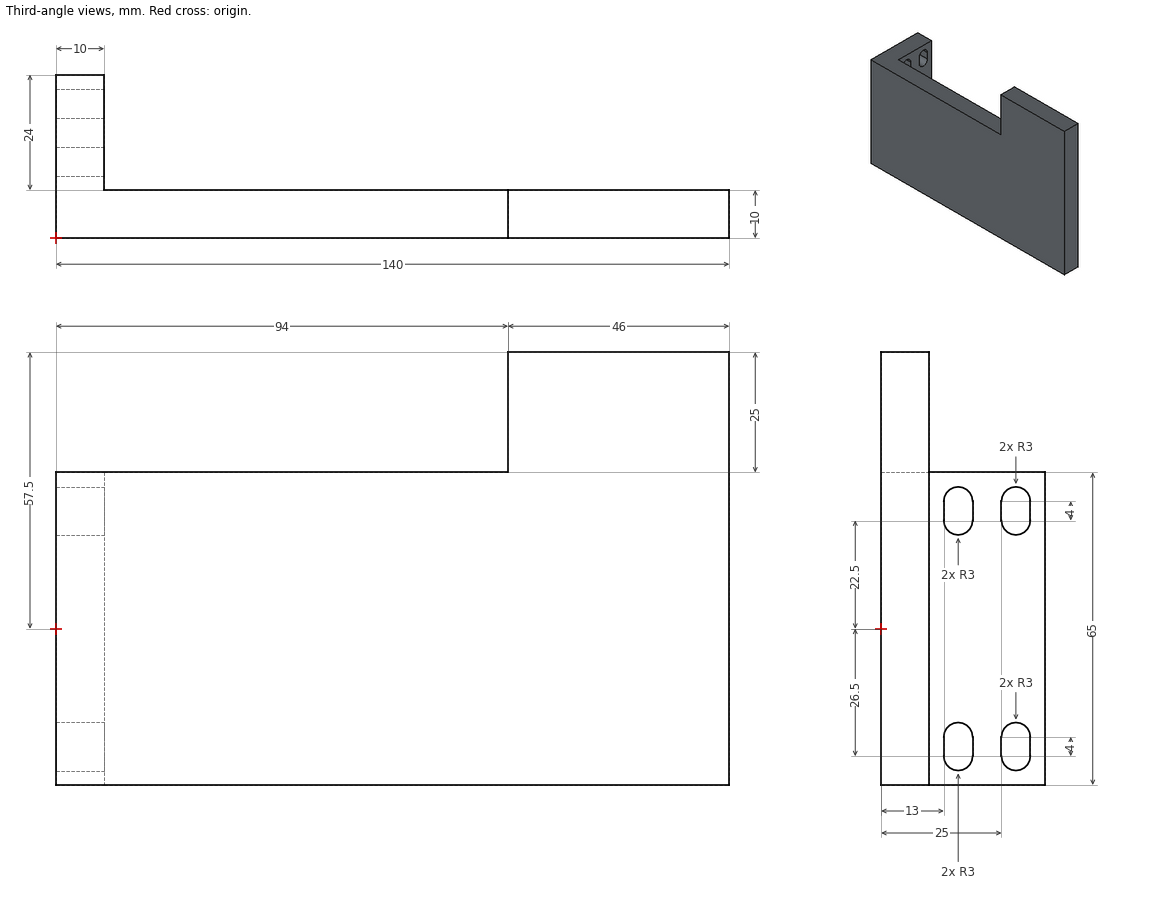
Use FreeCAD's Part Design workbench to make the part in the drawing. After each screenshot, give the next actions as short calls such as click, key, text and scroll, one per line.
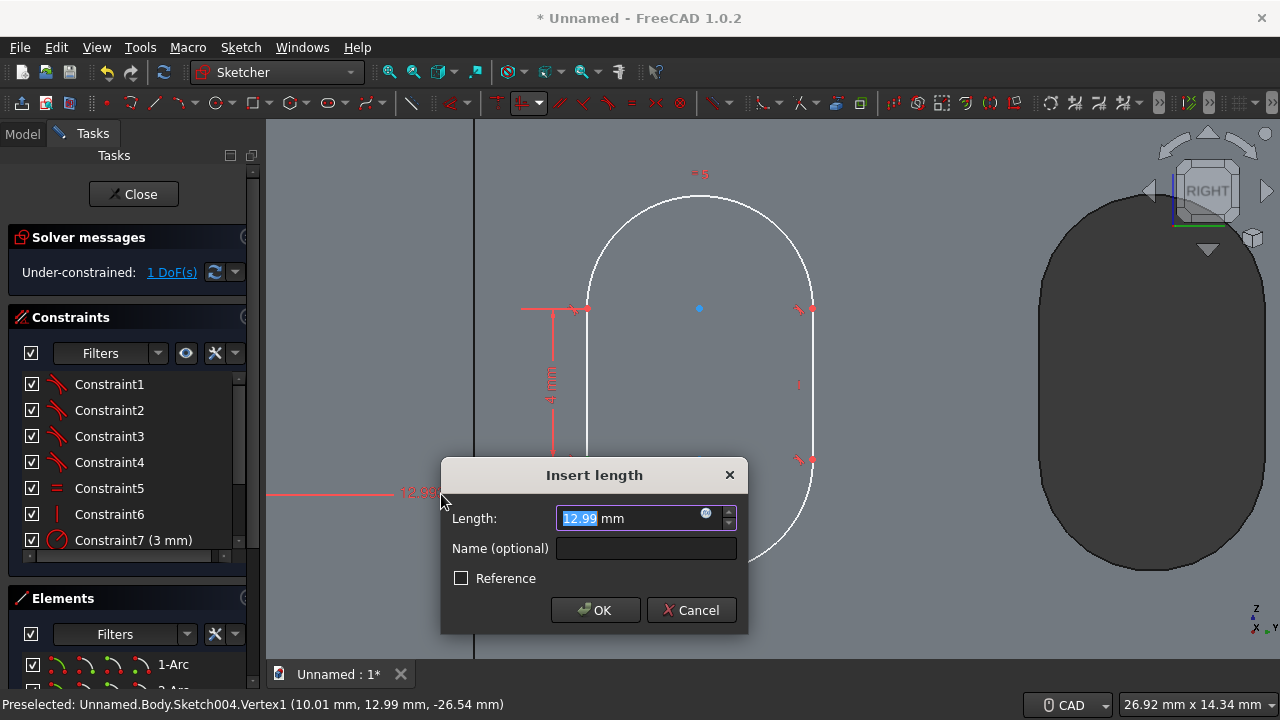
text(13)
key(Return)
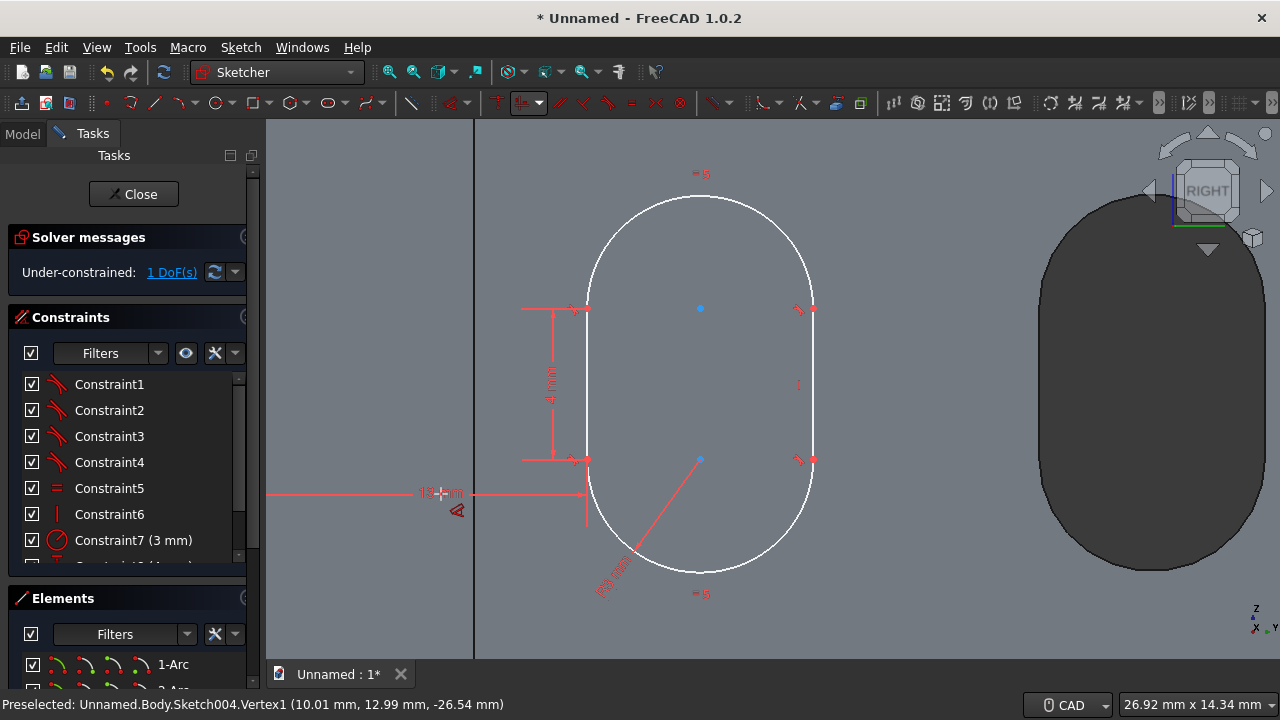
click(587, 460)
click(621, 303)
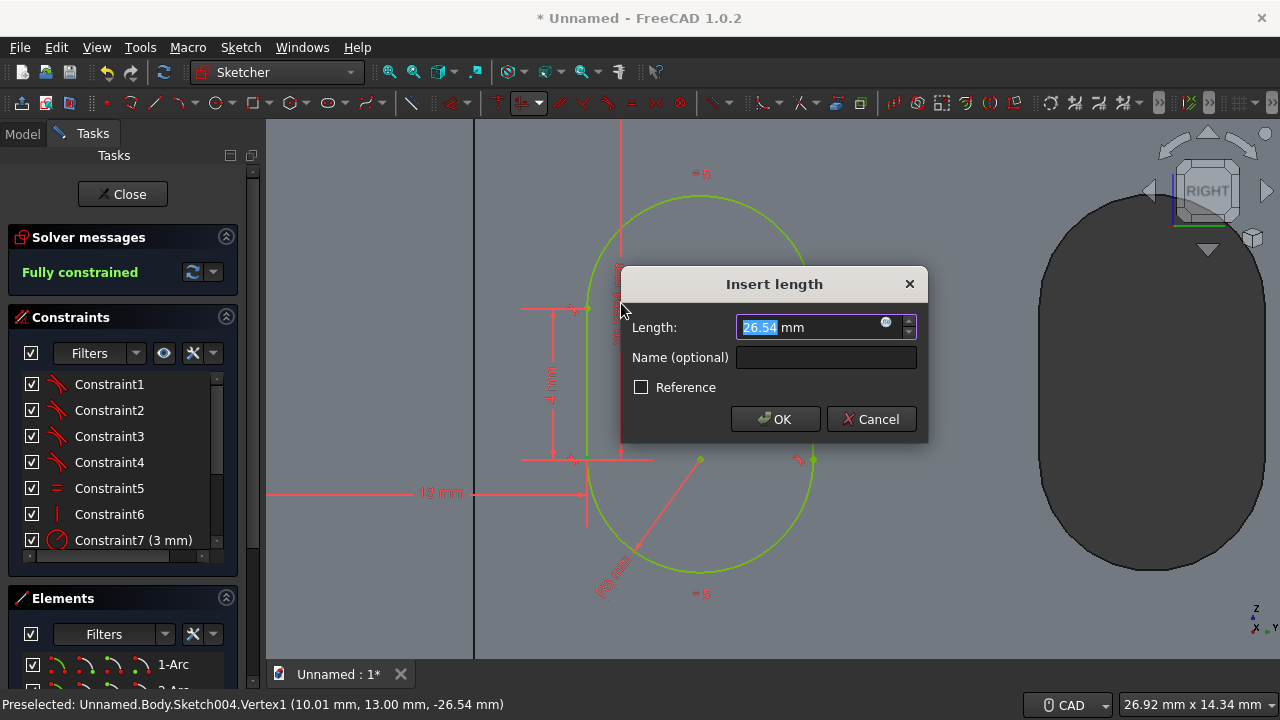
text(26.5)
key(Return)
key(Escape)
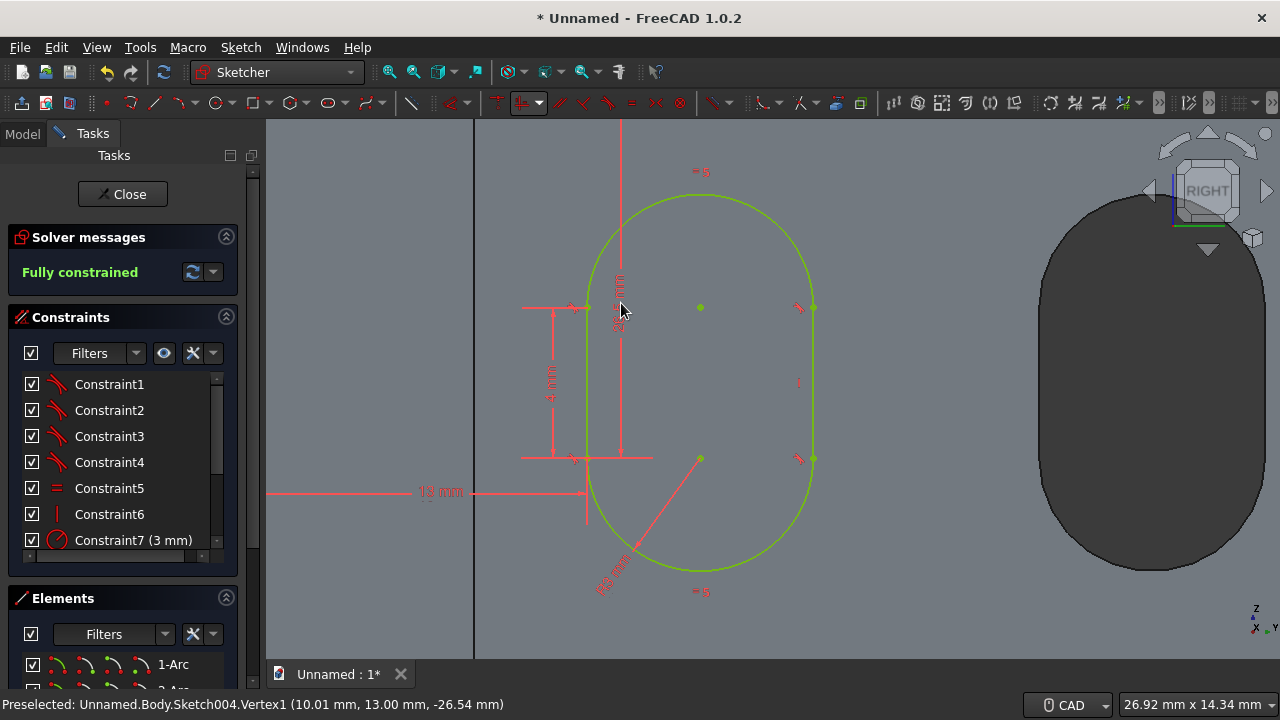
click(123, 194)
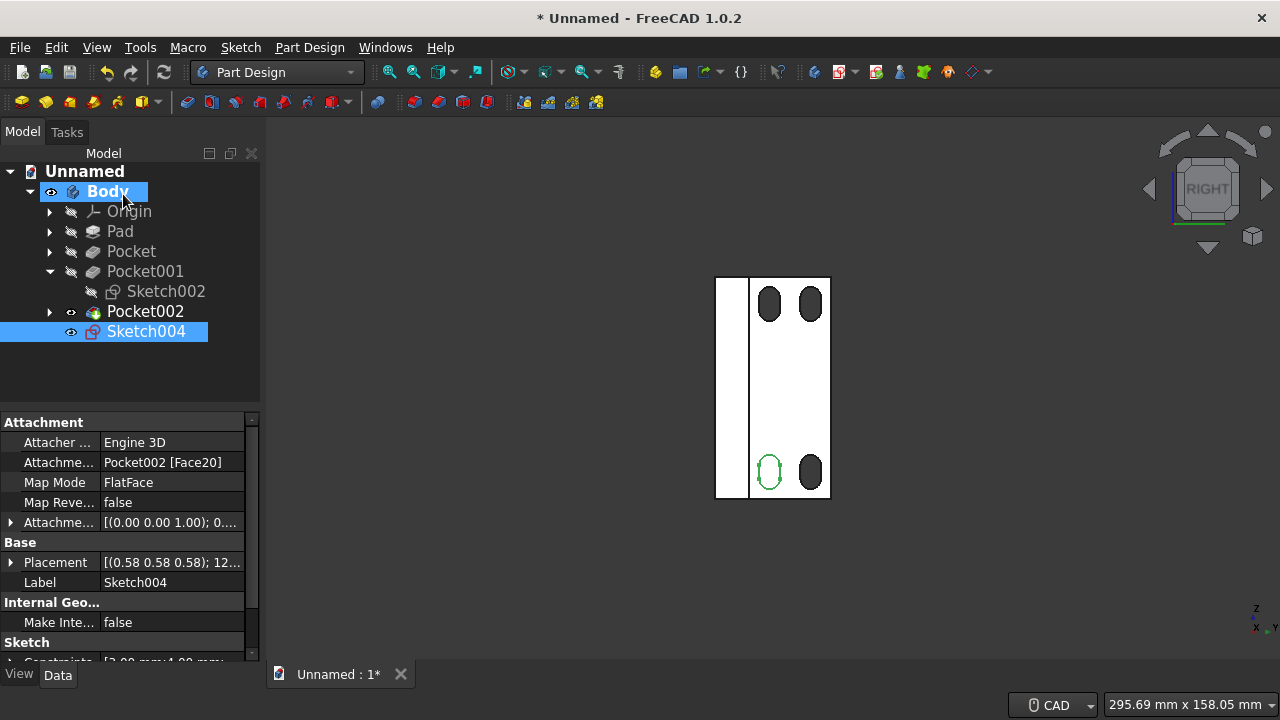
click(188, 102)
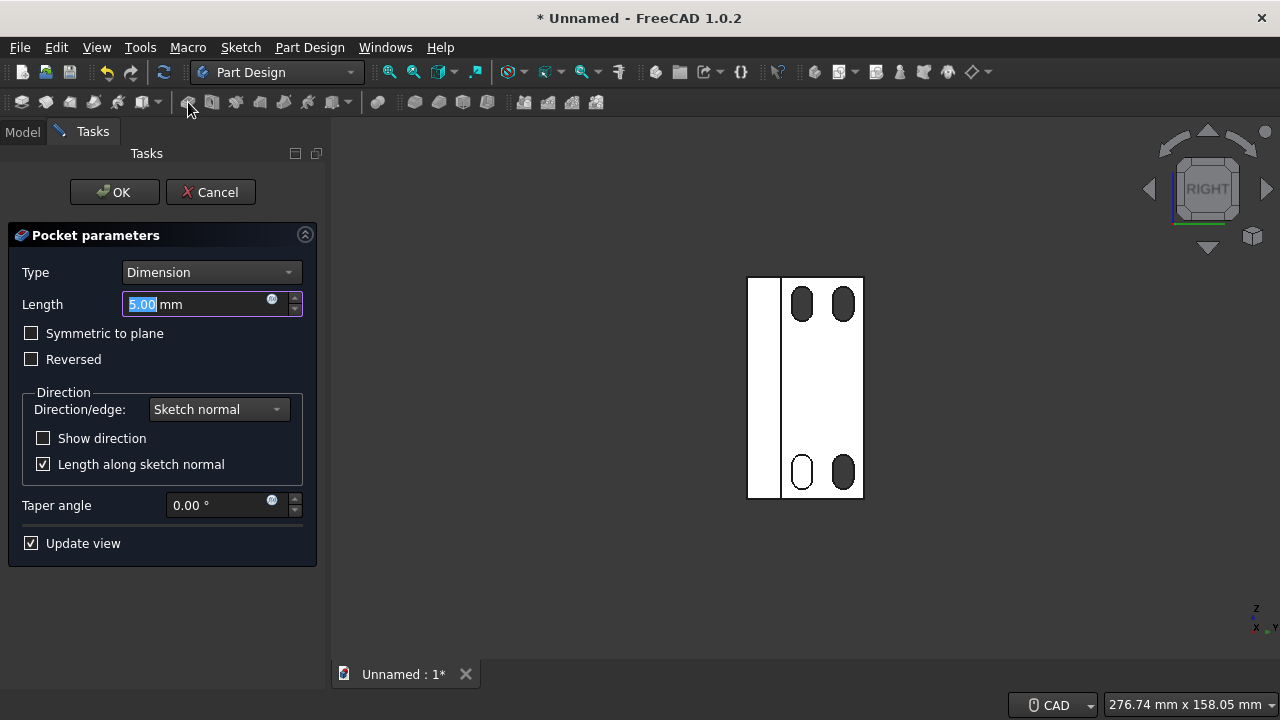
click(212, 272)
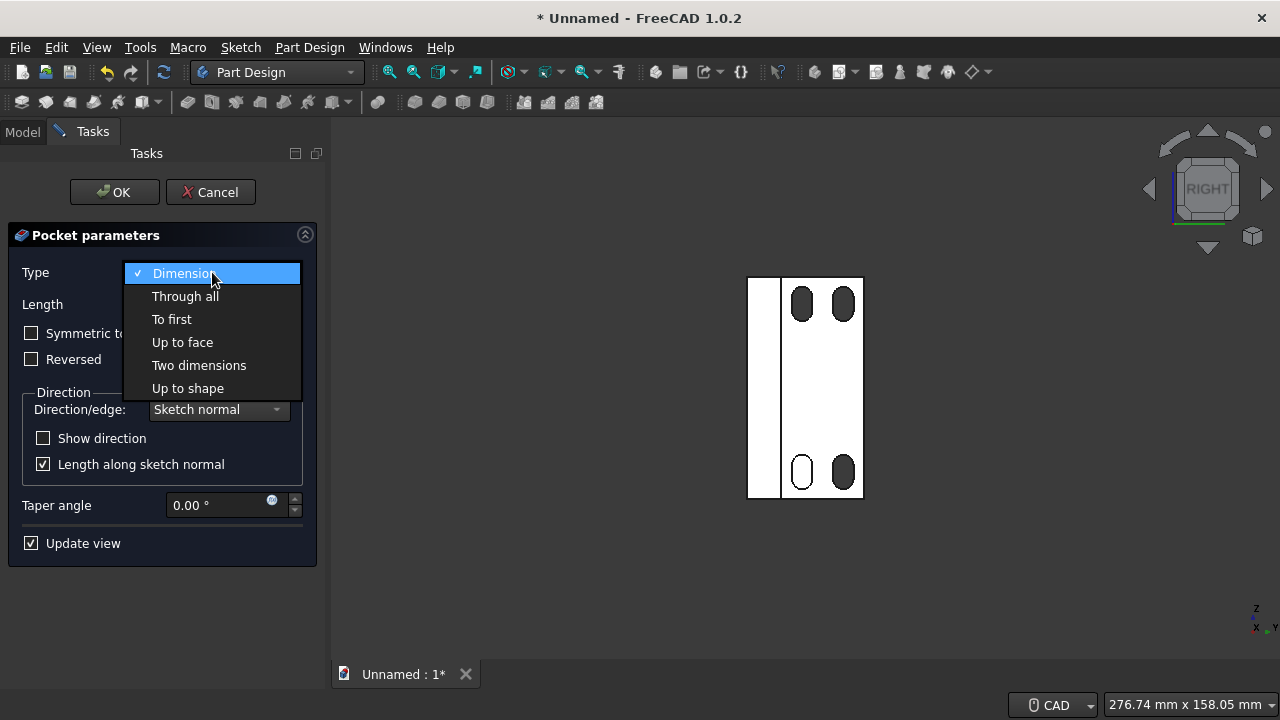
click(212, 320)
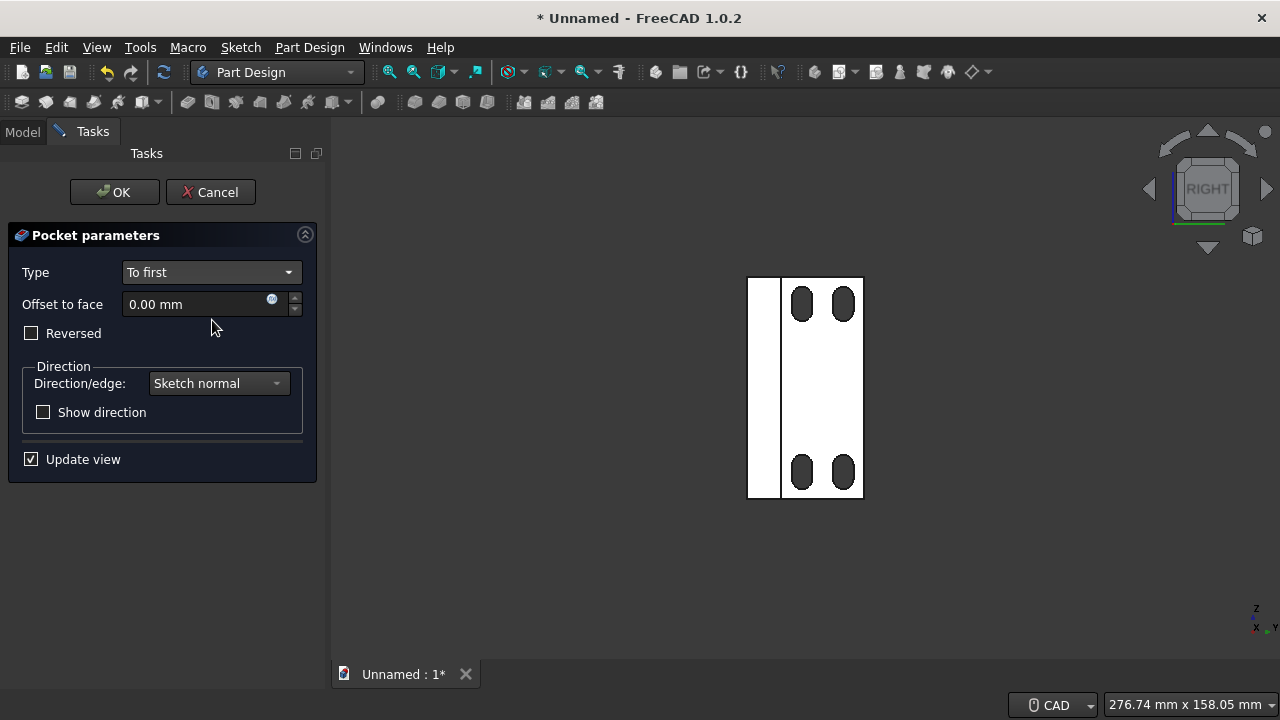
click(115, 192)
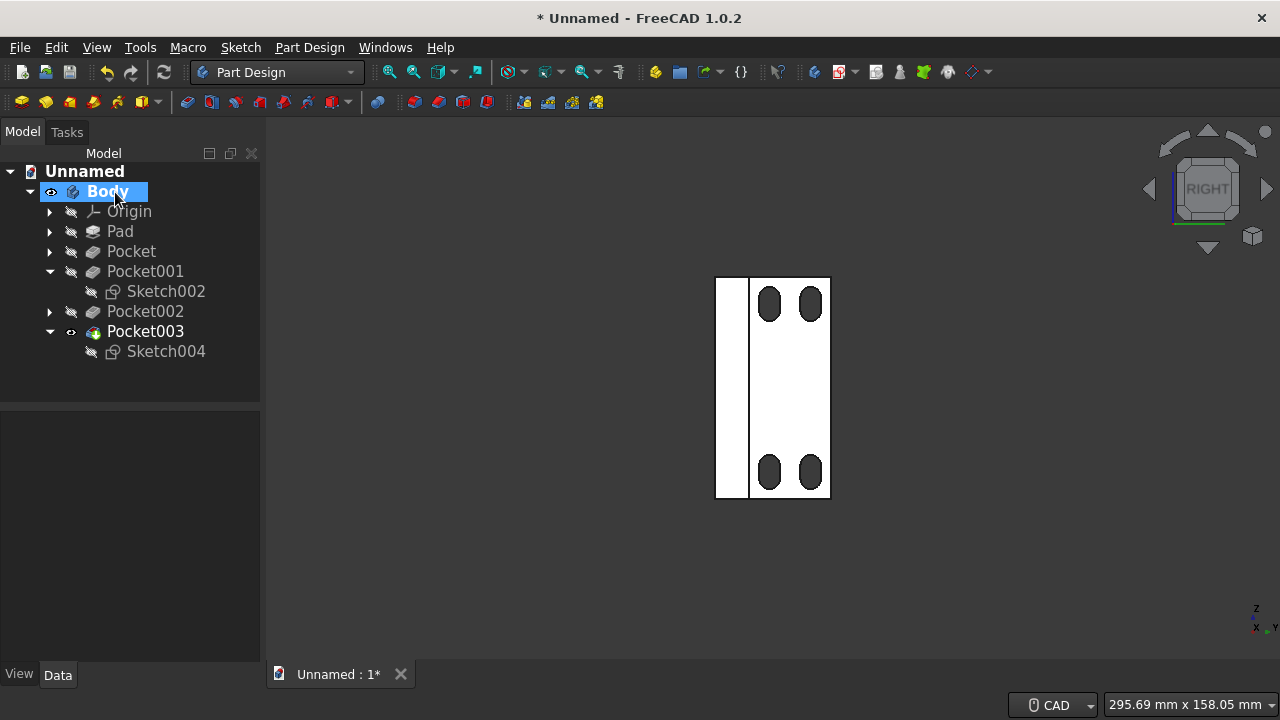
click(390, 72)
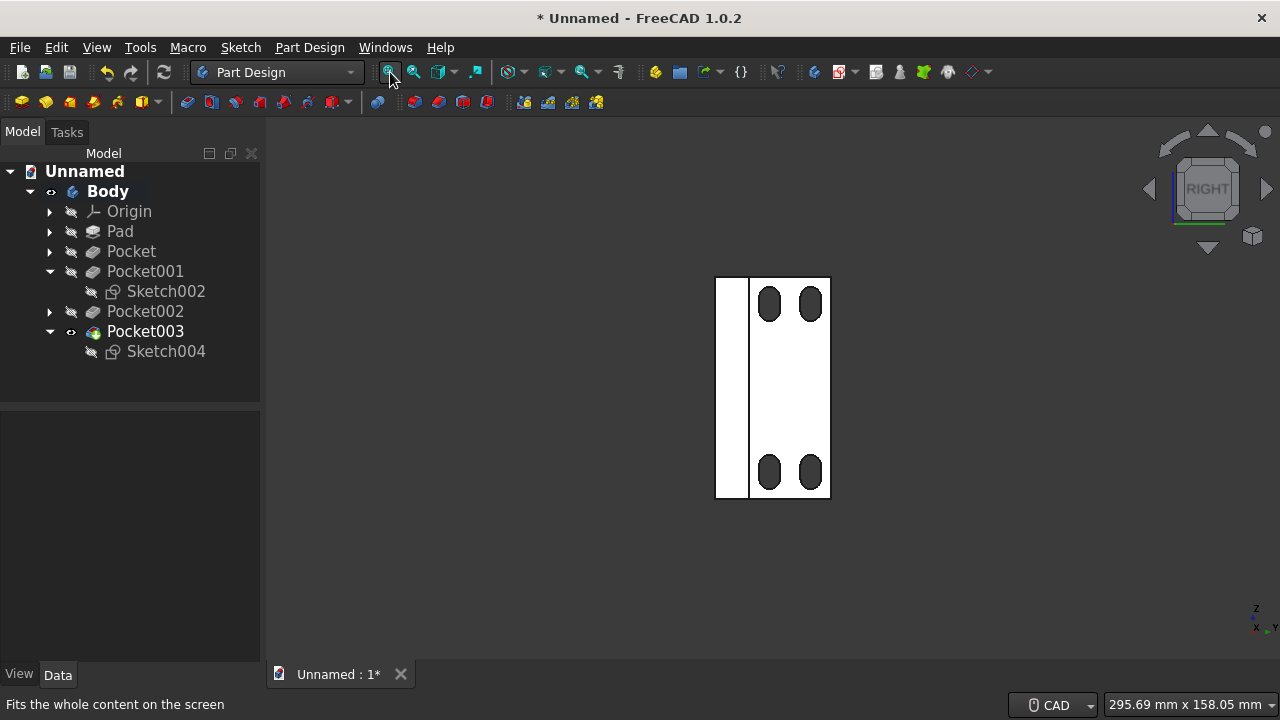
key(4)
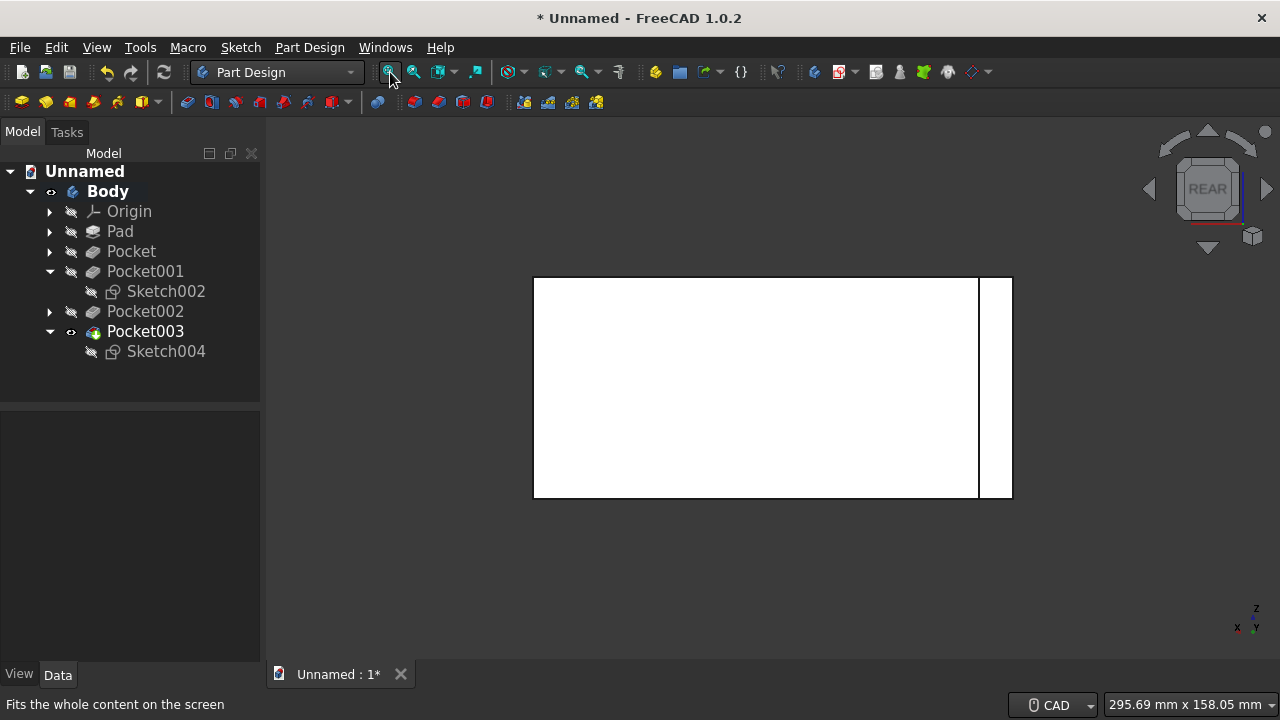
click(692, 387)